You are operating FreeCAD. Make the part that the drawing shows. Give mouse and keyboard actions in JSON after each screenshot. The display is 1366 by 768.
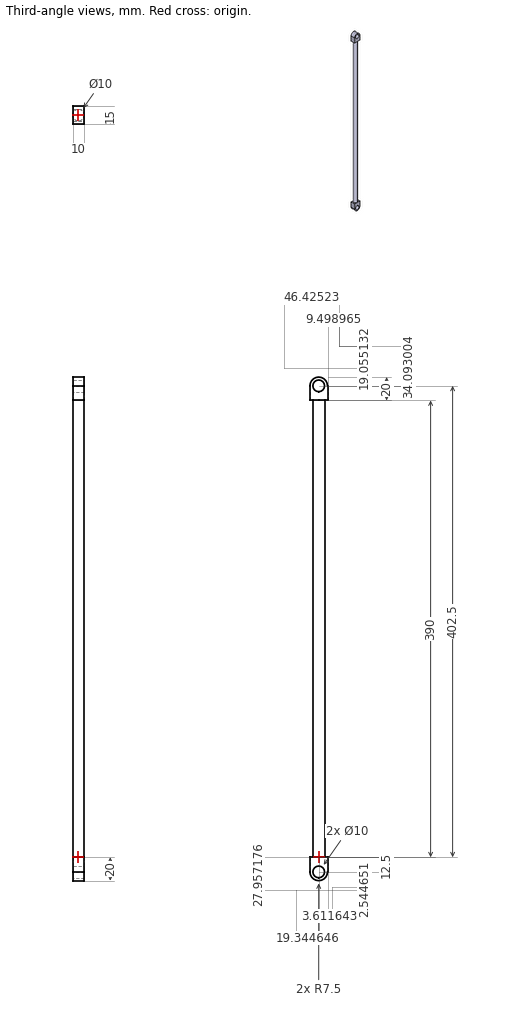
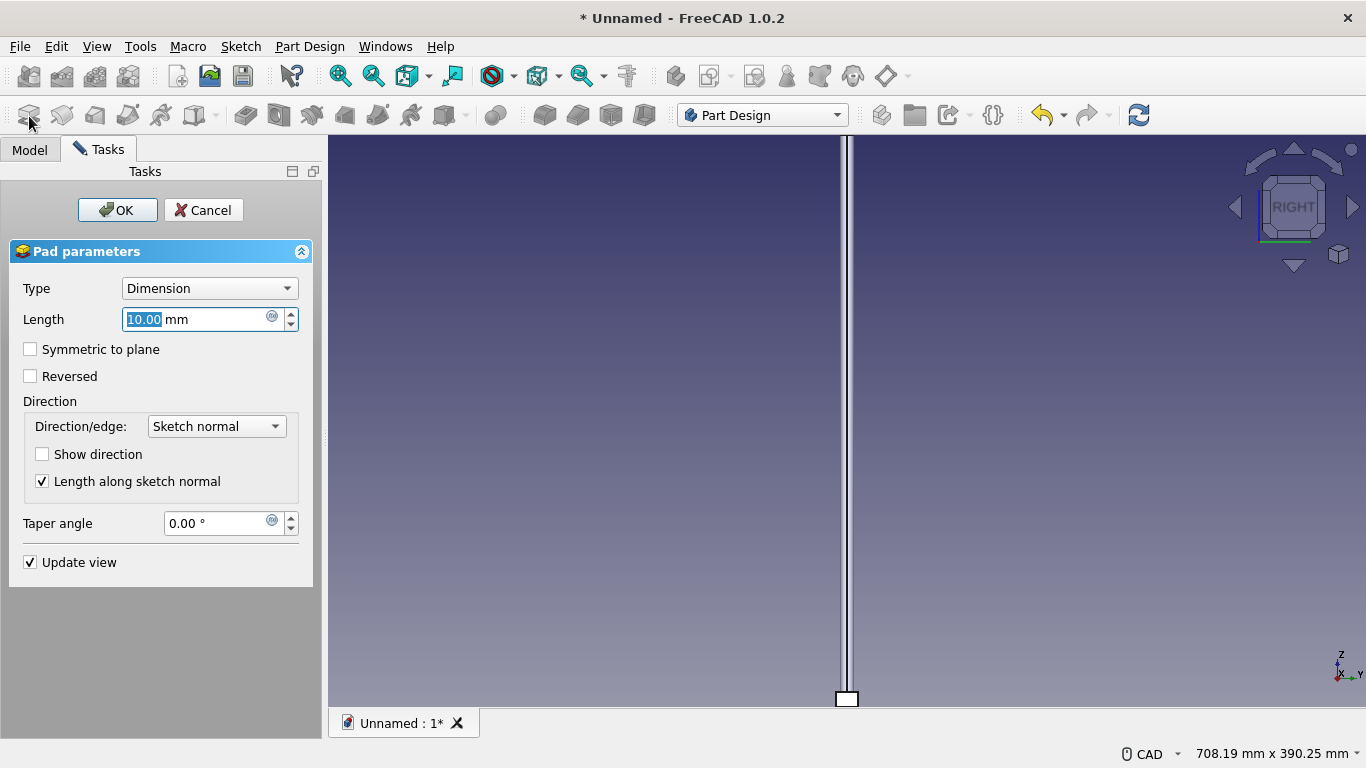
{"action": "type", "text": "20"}
{"action": "key", "text": "Tab"}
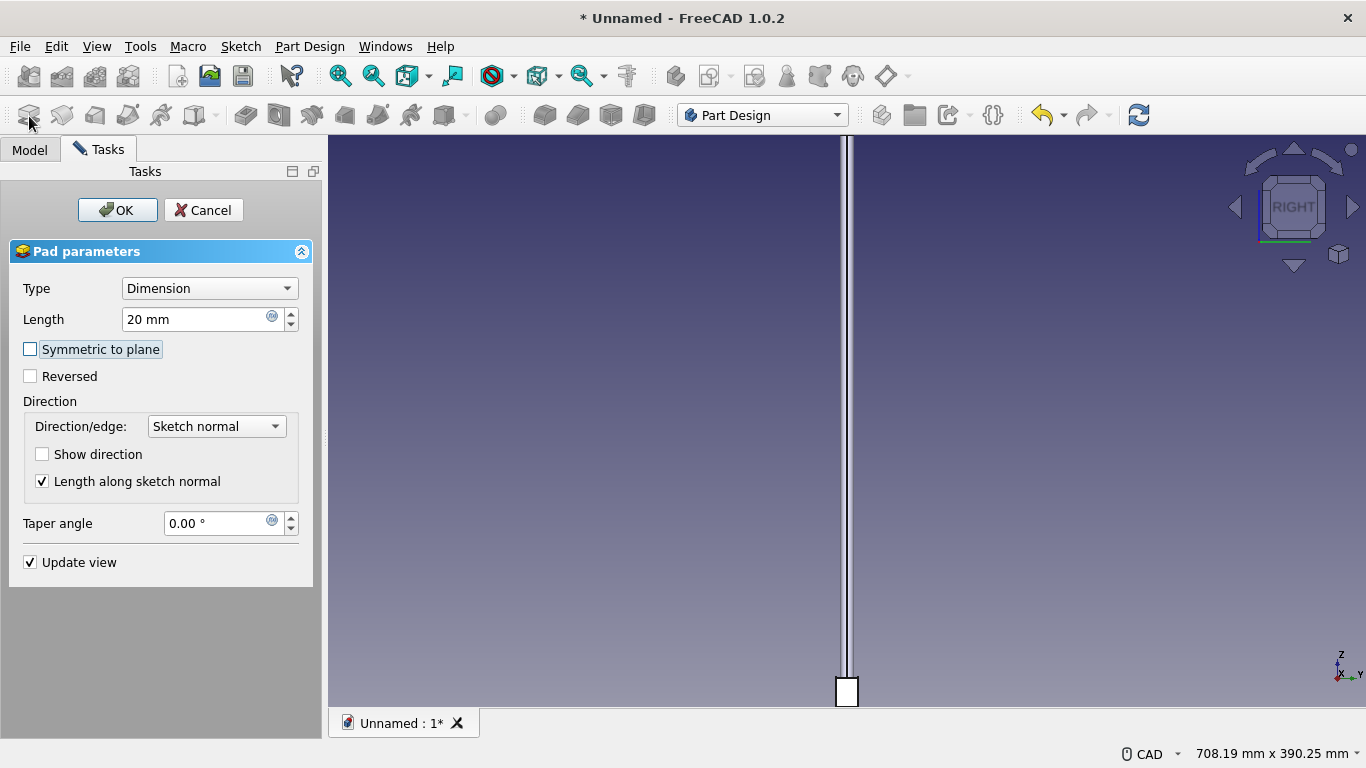
{"action": "left_click", "coordinate": [31, 376]}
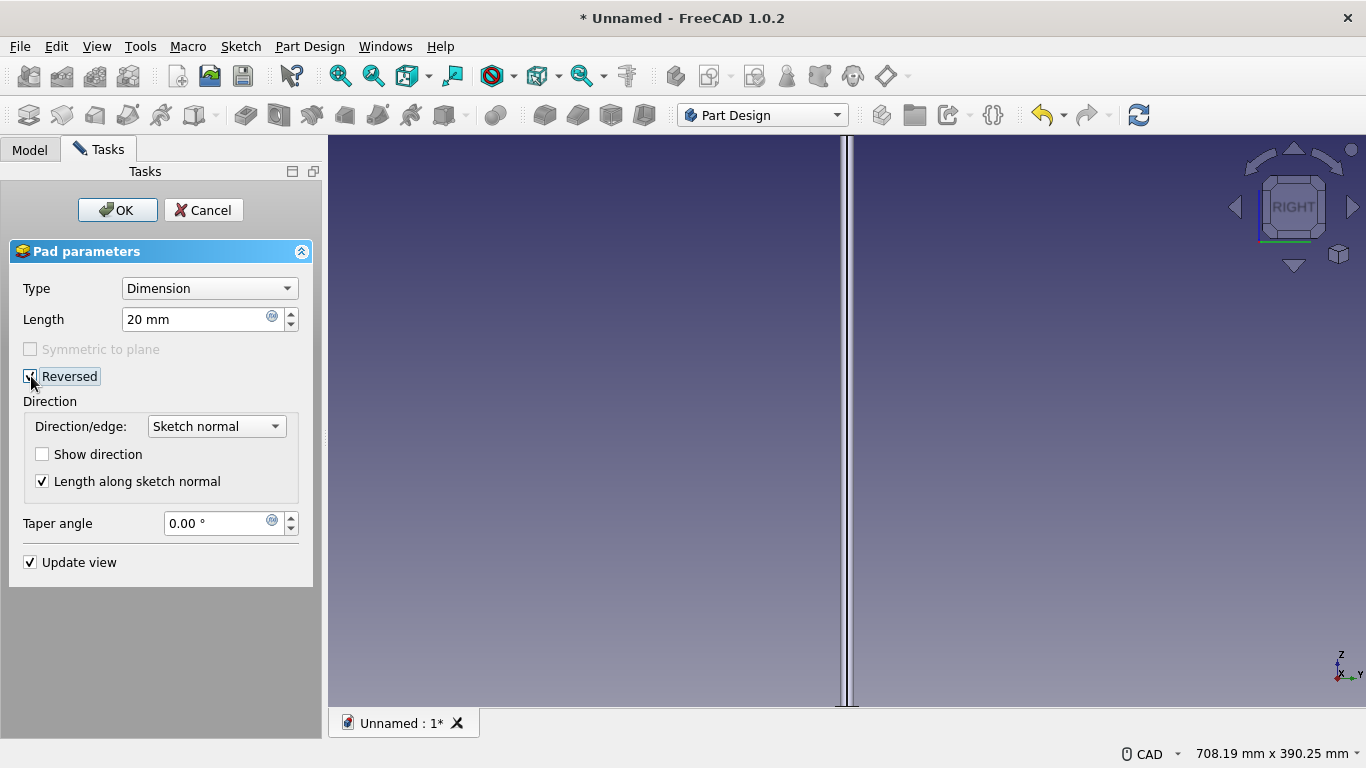
{"action": "left_click", "coordinate": [118, 210]}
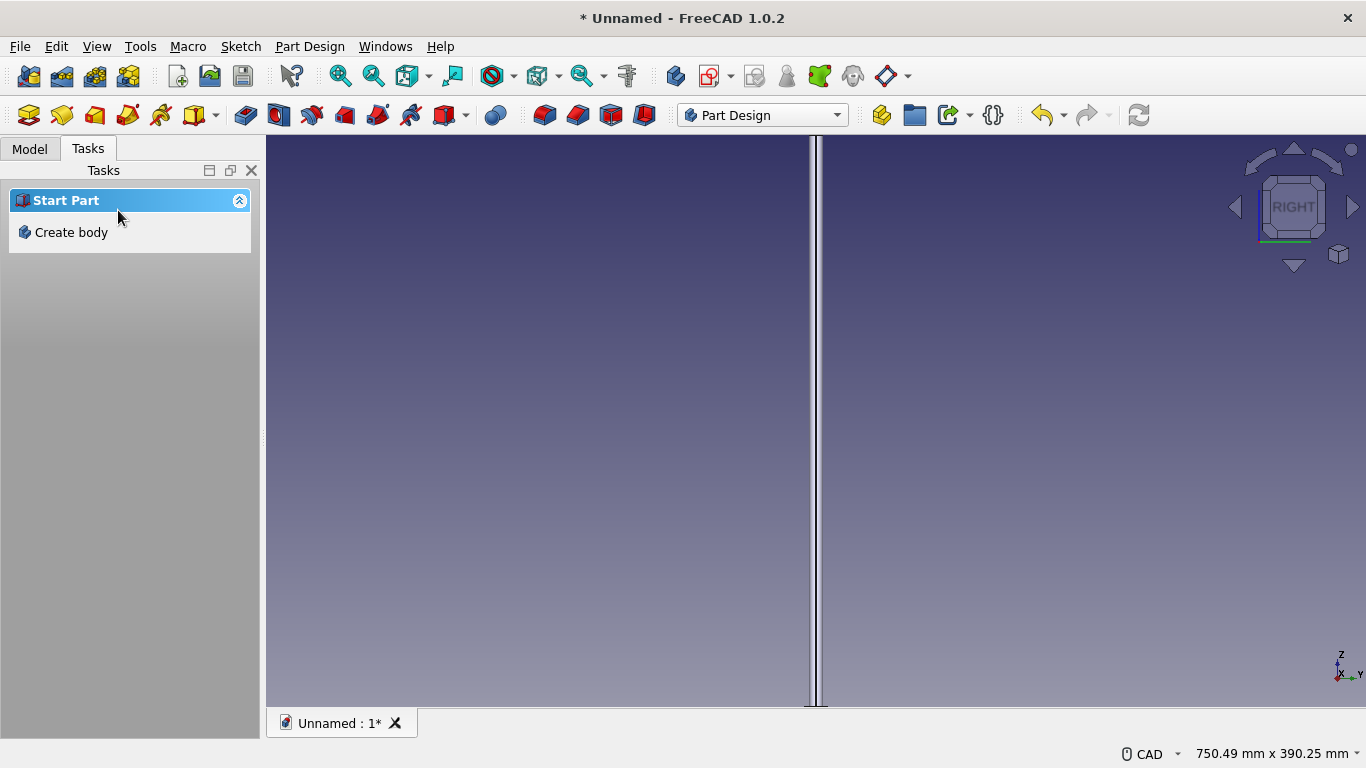
{"action": "left_click", "coordinate": [341, 76]}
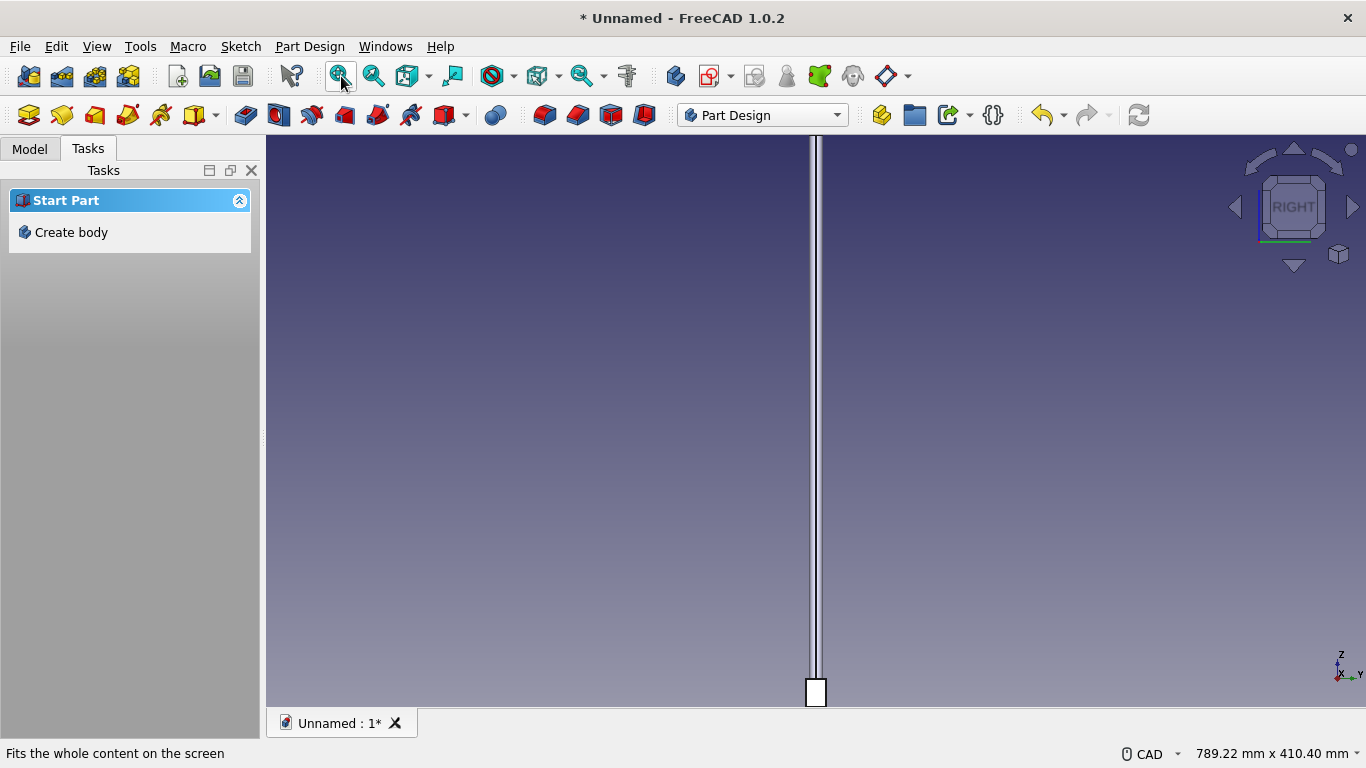
{"action": "key", "text": "0"}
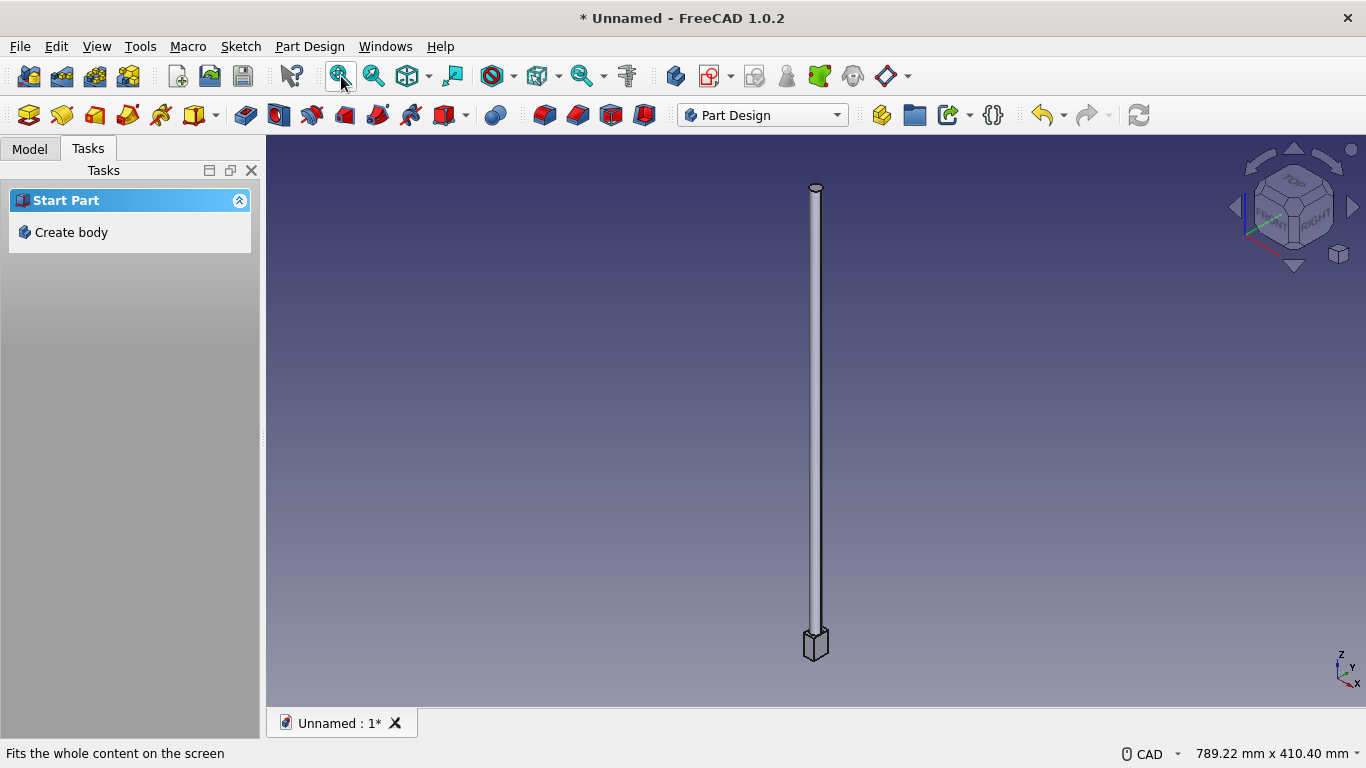
{"action": "scroll", "coordinate": [816, 187], "scroll_direction": "up", "scroll_amount": 3}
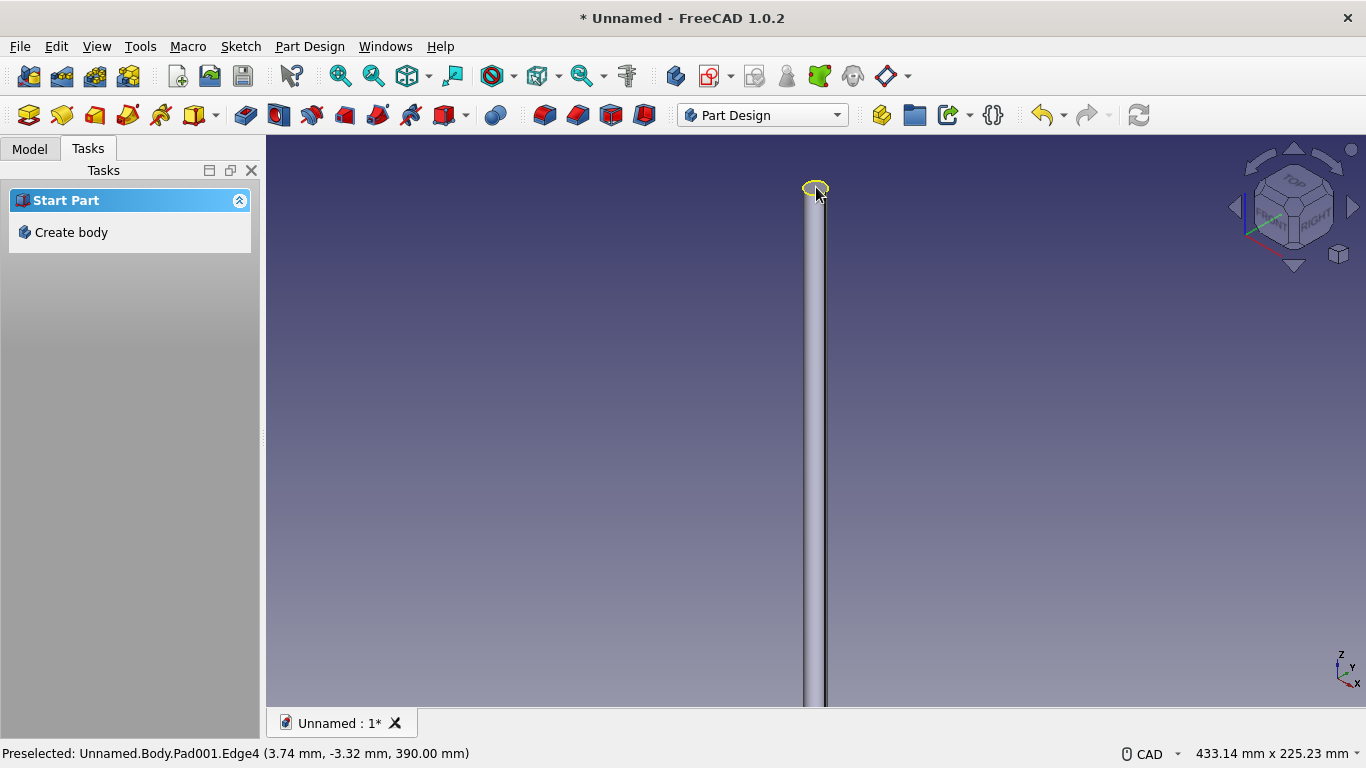
{"action": "left_click", "coordinate": [341, 76]}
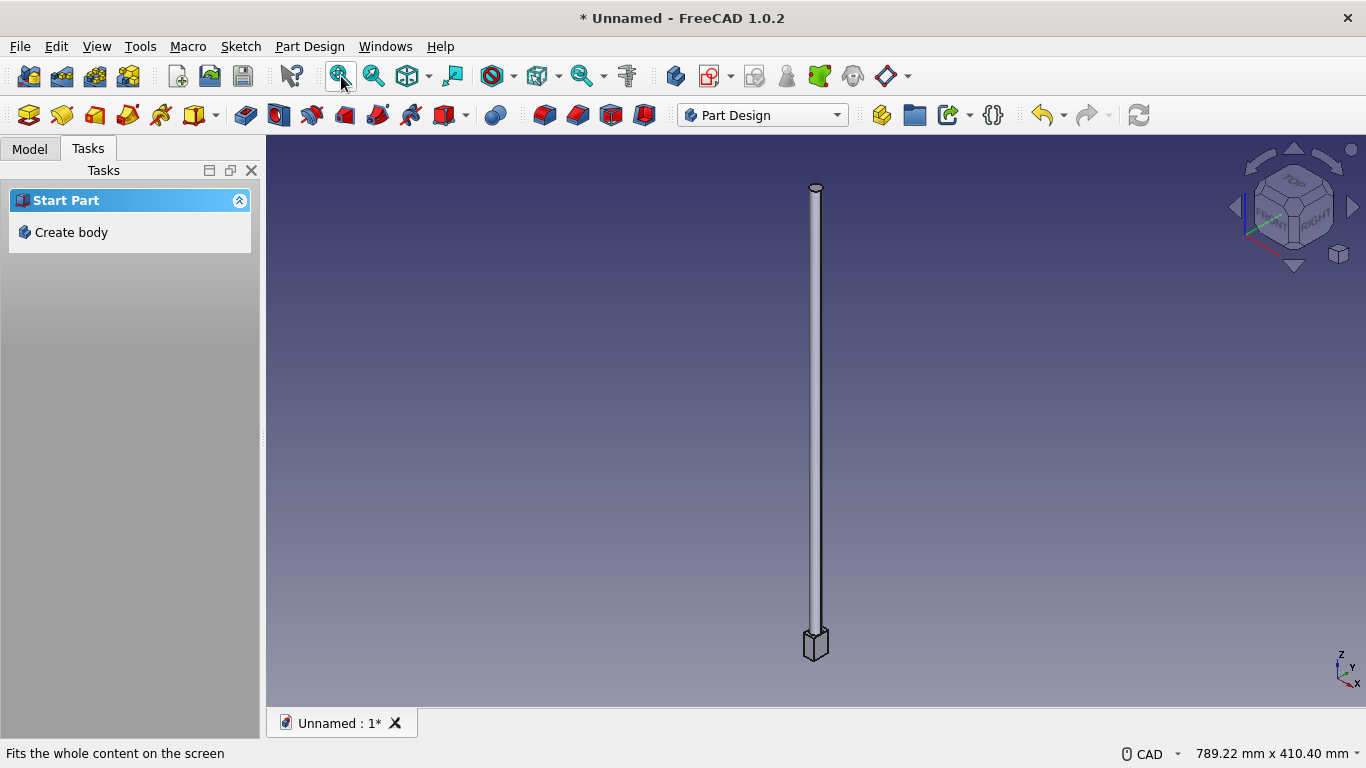
{"action": "key", "text": "2"}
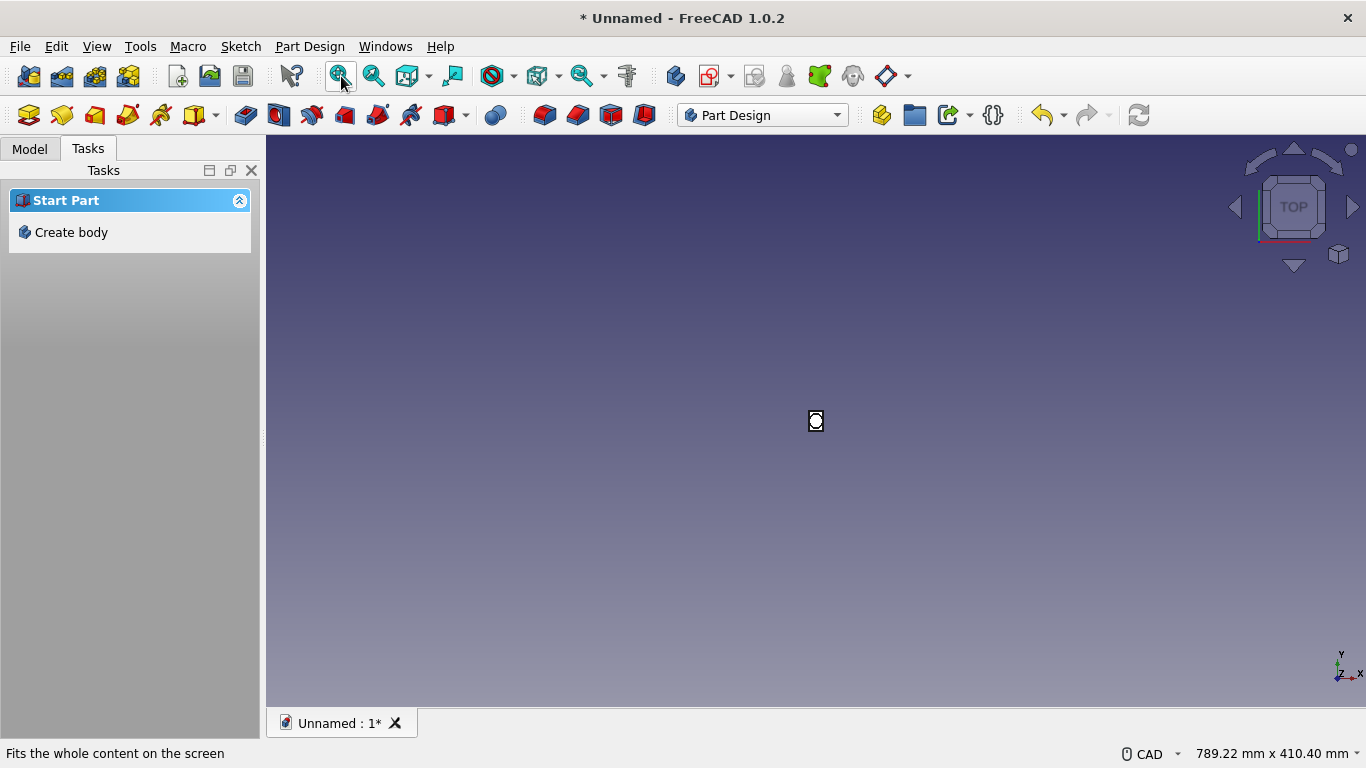
{"action": "left_click", "coordinate": [341, 76]}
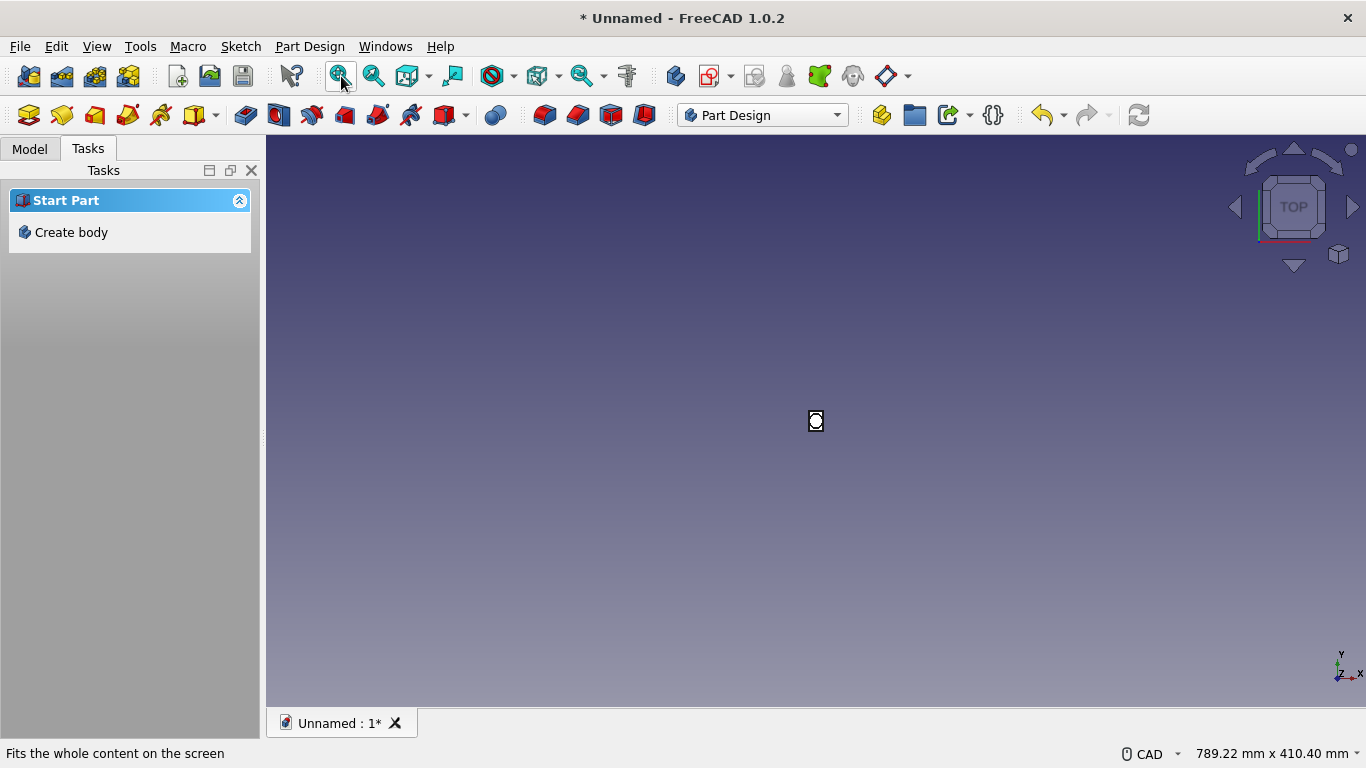
{"action": "scroll", "coordinate": [816, 420], "scroll_direction": "up", "scroll_amount": 3}